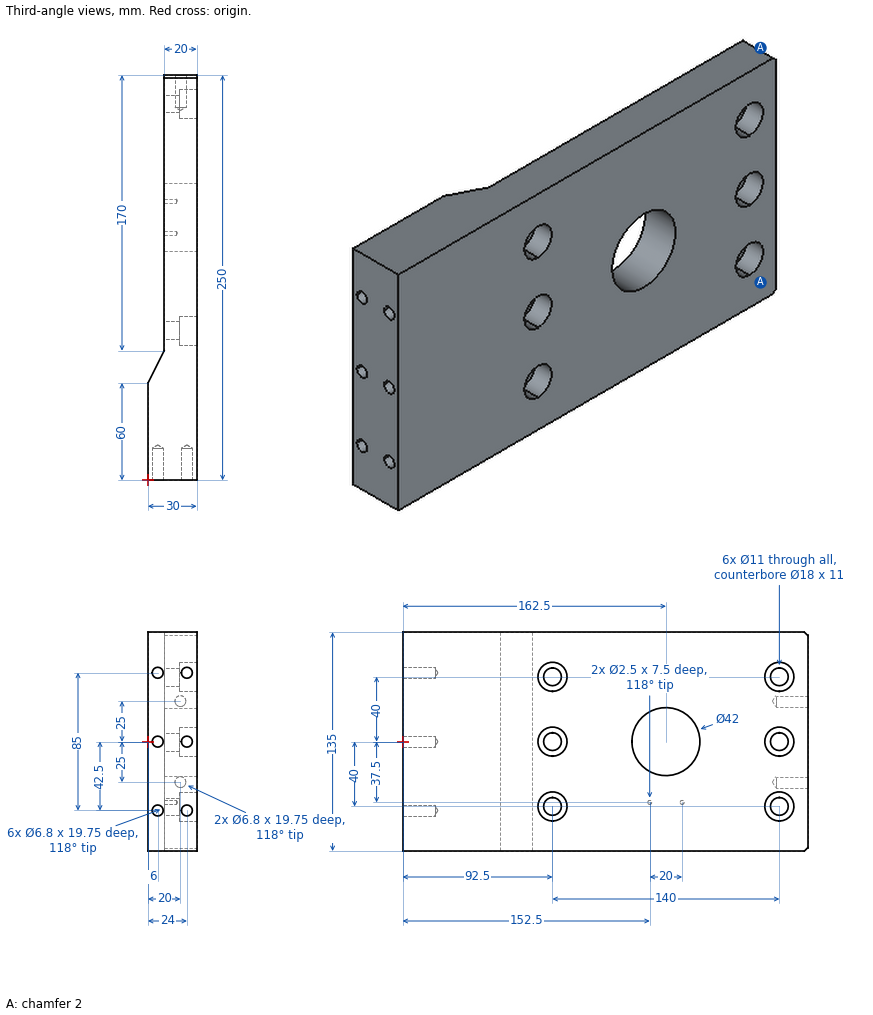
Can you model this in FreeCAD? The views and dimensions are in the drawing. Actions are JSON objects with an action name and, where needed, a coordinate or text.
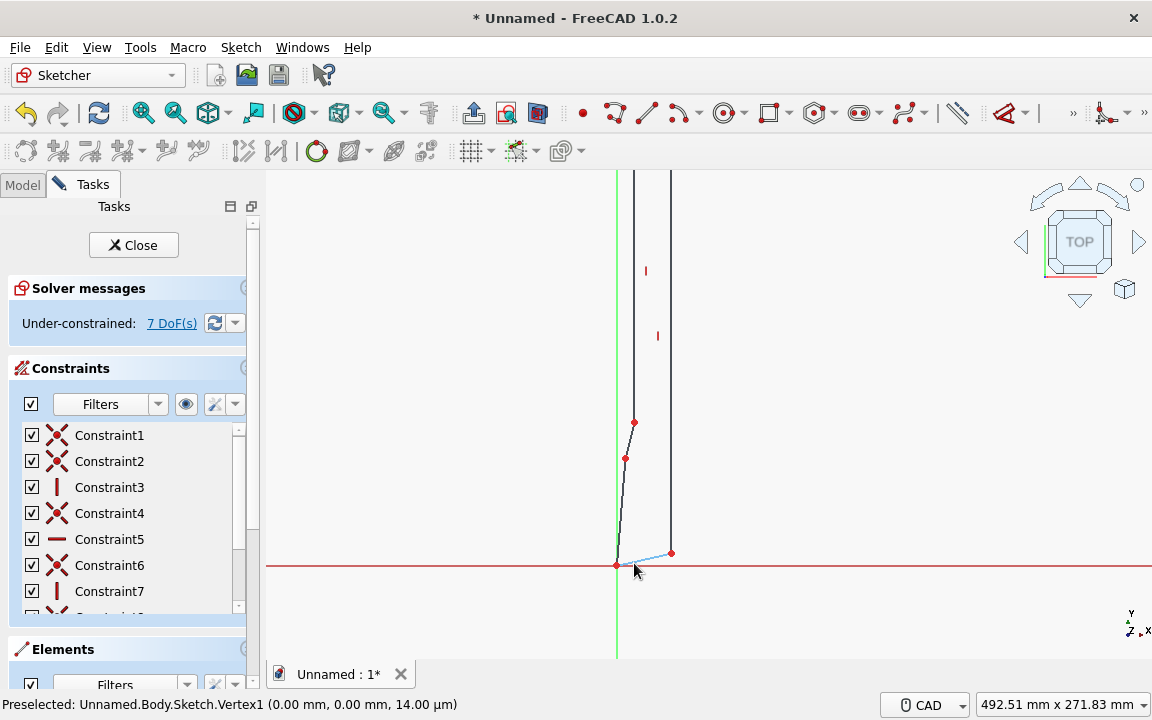
{"action": "left_click", "coordinate": [633, 562]}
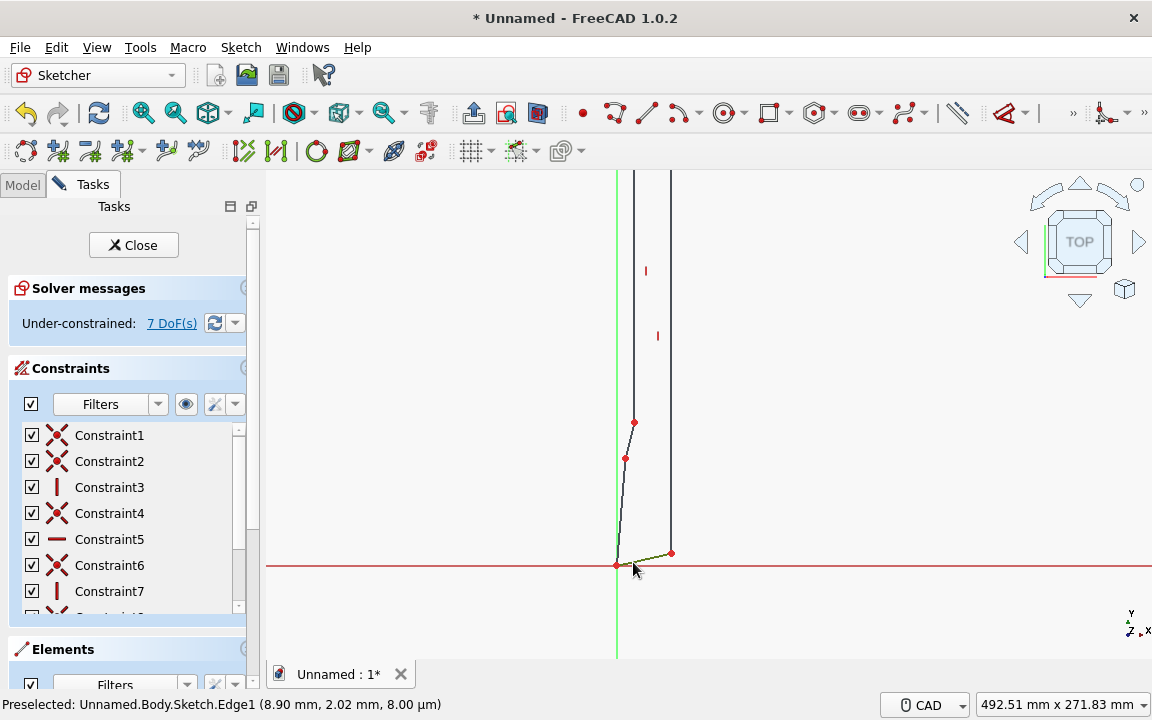
{"action": "key", "text": "h"}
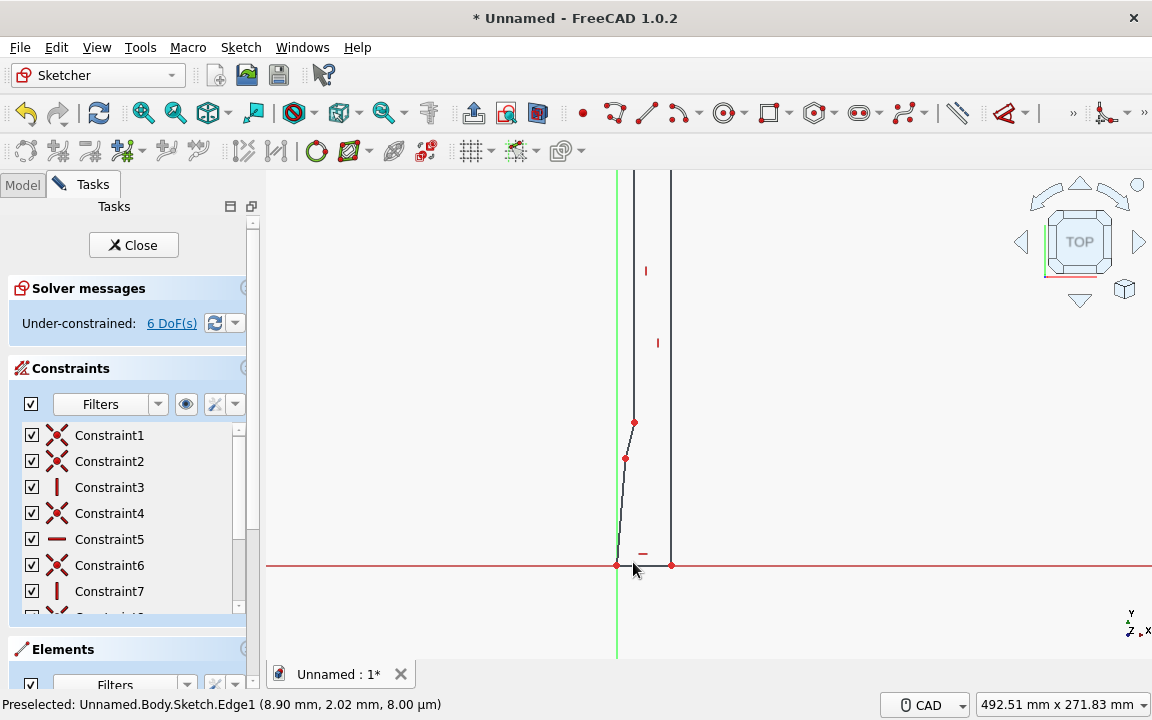
{"action": "left_click", "coordinate": [619, 534]}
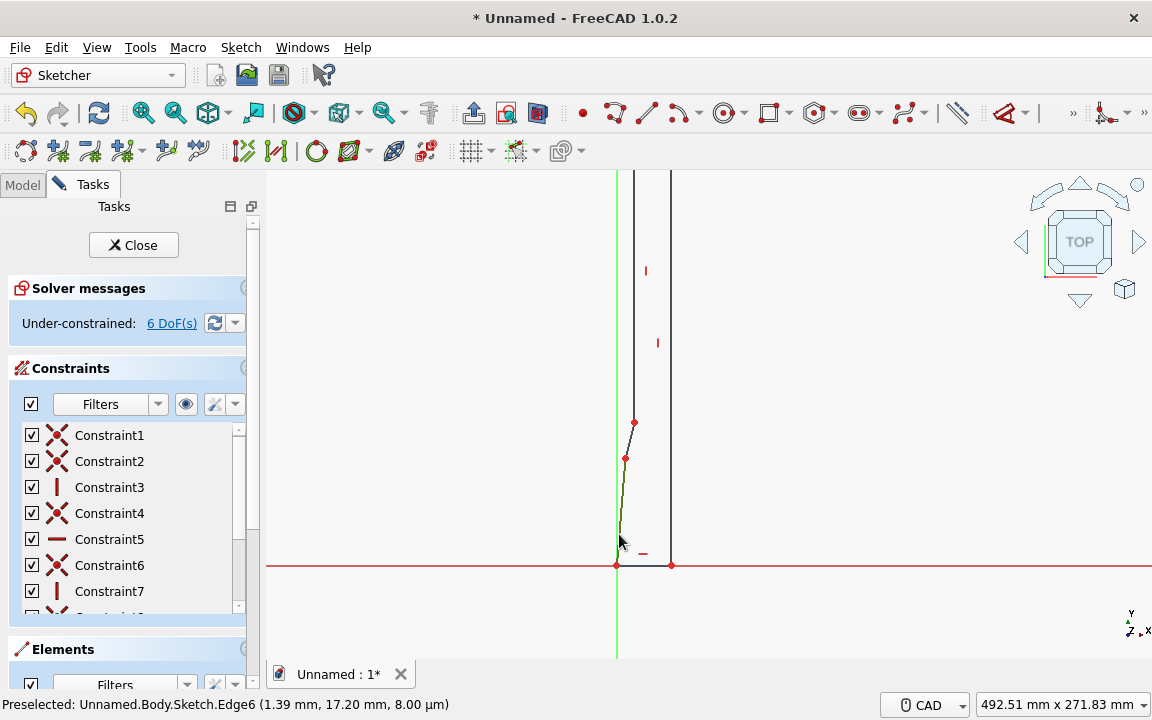
{"action": "key", "text": "v"}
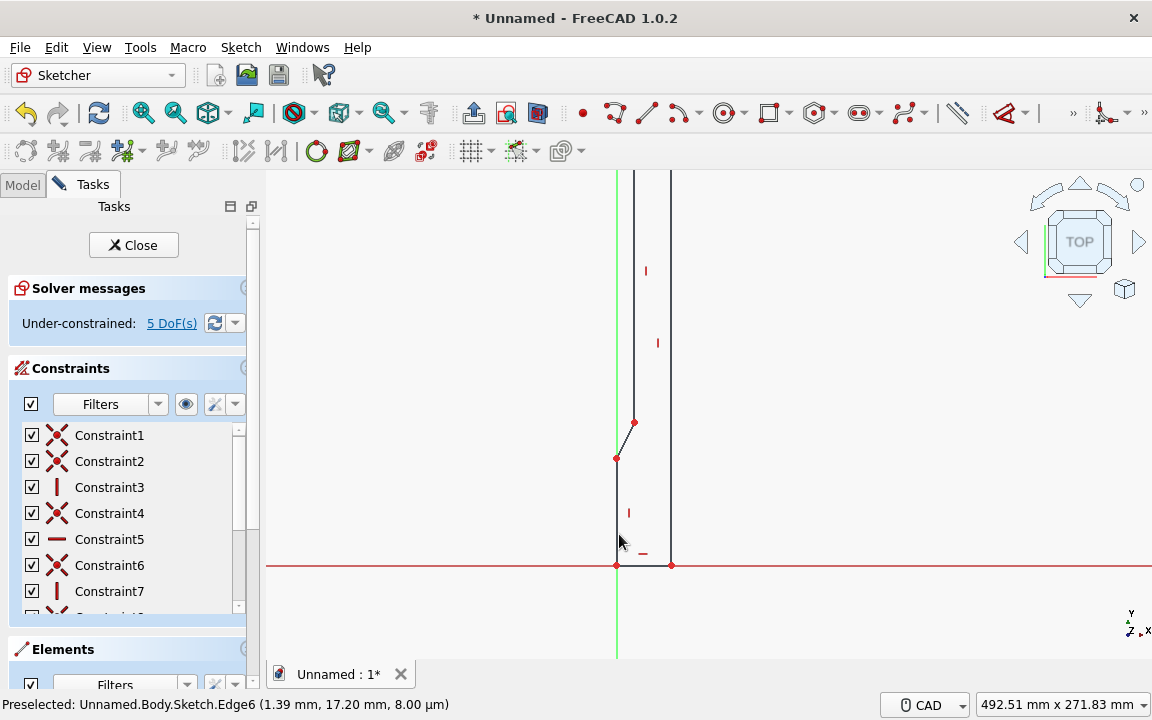
{"action": "left_click", "coordinate": [1004, 114]}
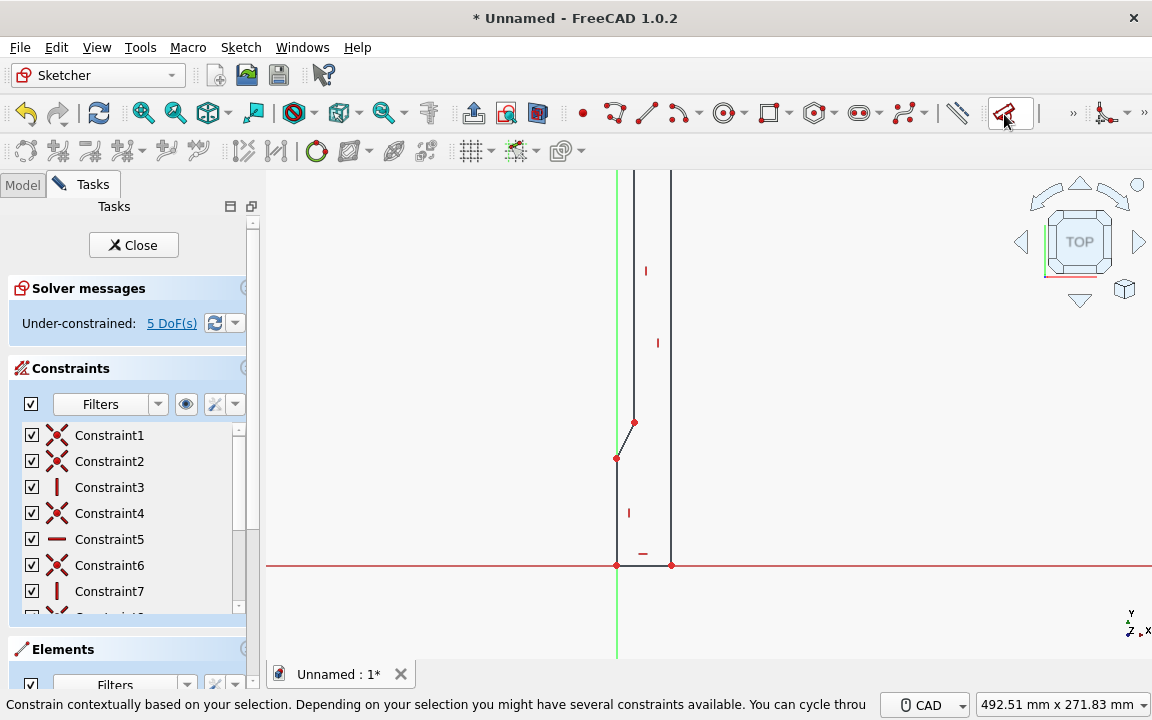
{"action": "left_click", "coordinate": [633, 566]}
{"action": "left_click", "coordinate": [644, 600]}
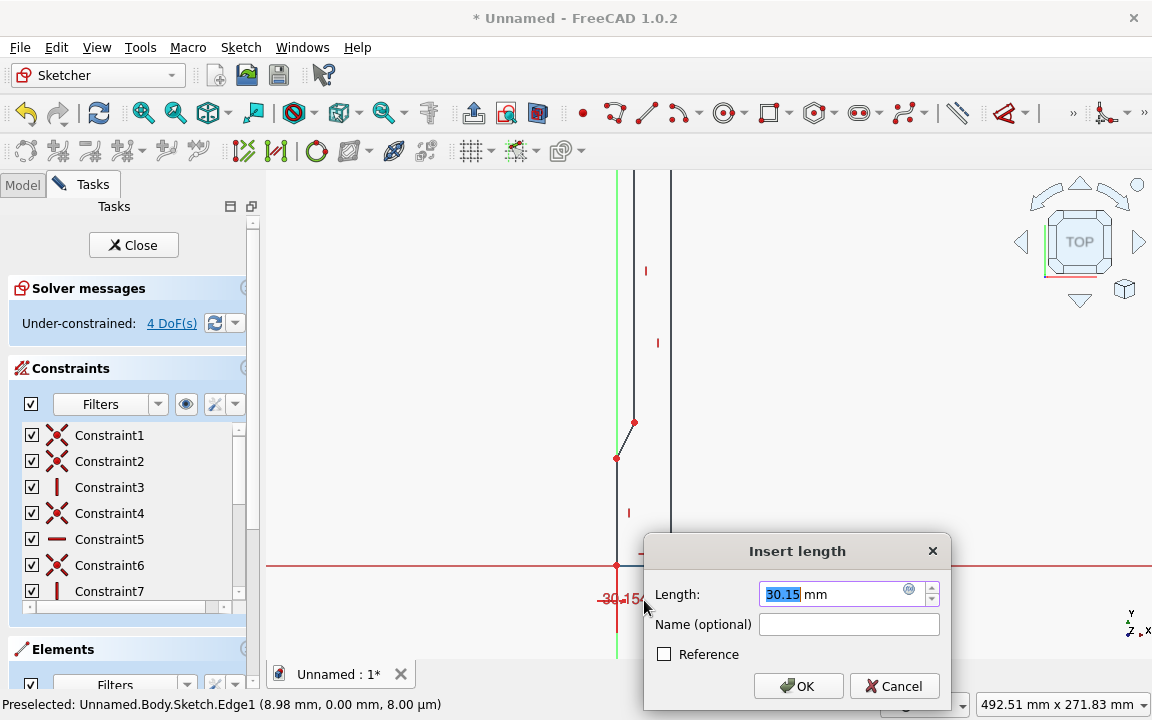
{"action": "type", "text": "30"}
{"action": "key", "text": "Return"}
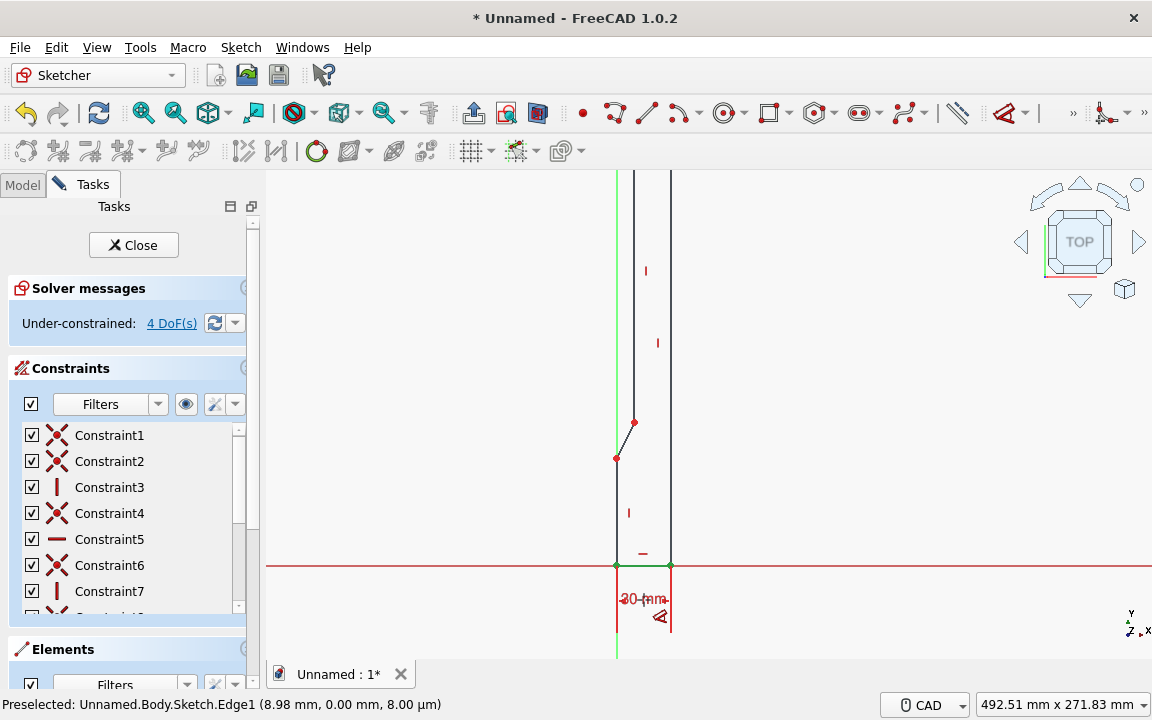
{"action": "scroll", "coordinate": [634, 564], "scroll_direction": "down", "scroll_amount": 2}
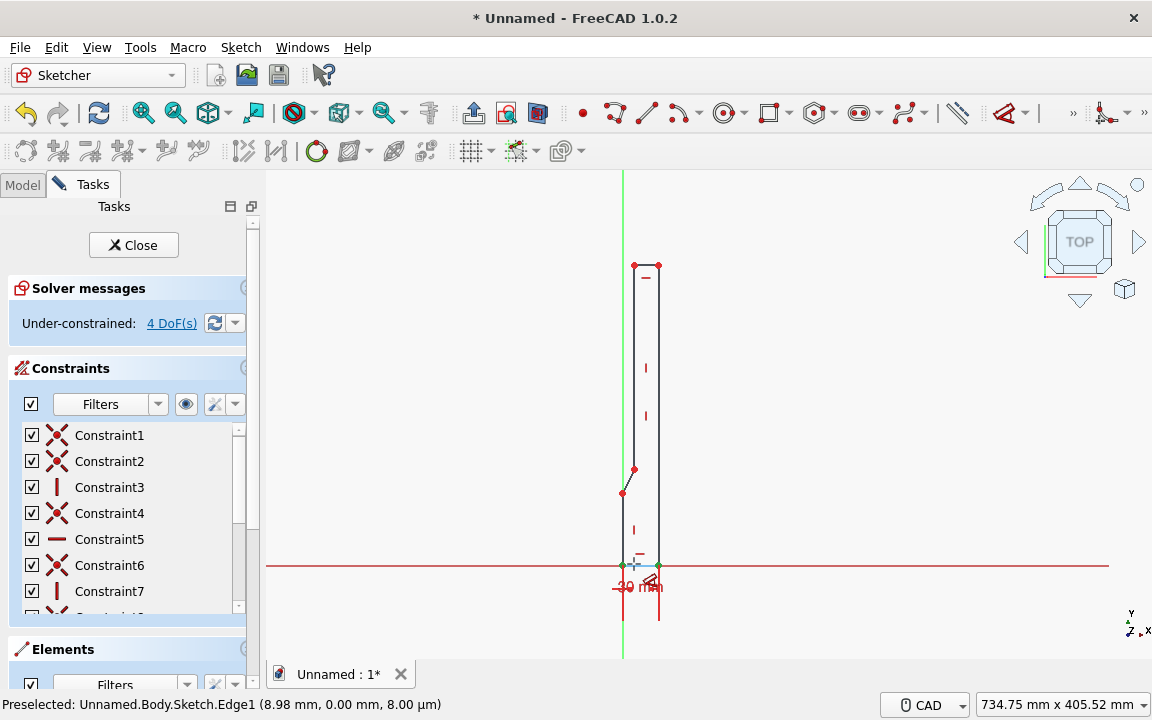
{"action": "scroll", "coordinate": [652, 265], "scroll_direction": "up", "scroll_amount": 4}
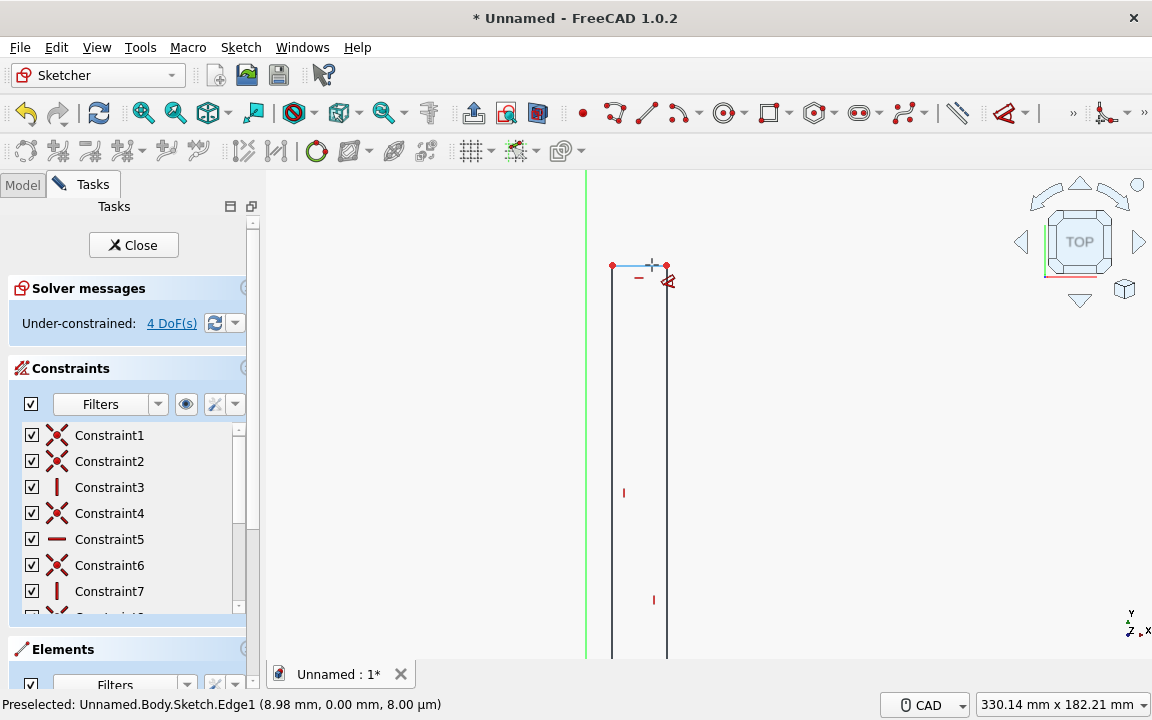
{"action": "left_click", "coordinate": [650, 266]}
{"action": "left_click", "coordinate": [640, 232]}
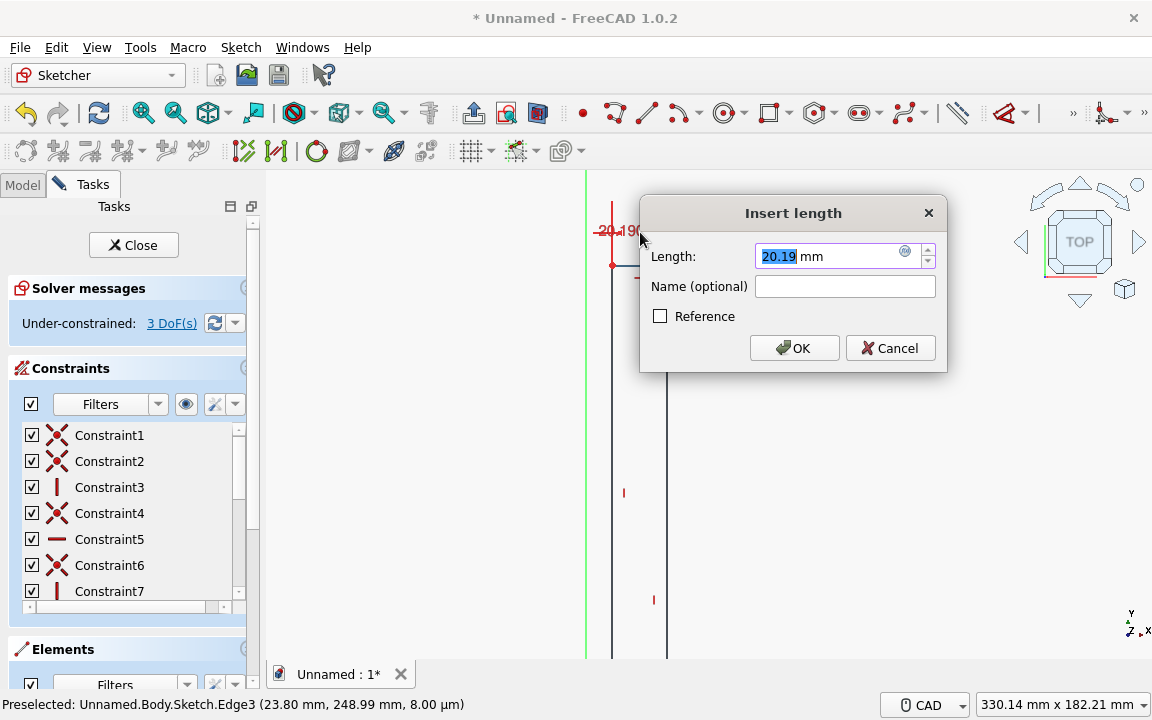
{"action": "type", "text": "20"}
{"action": "key", "text": "Return"}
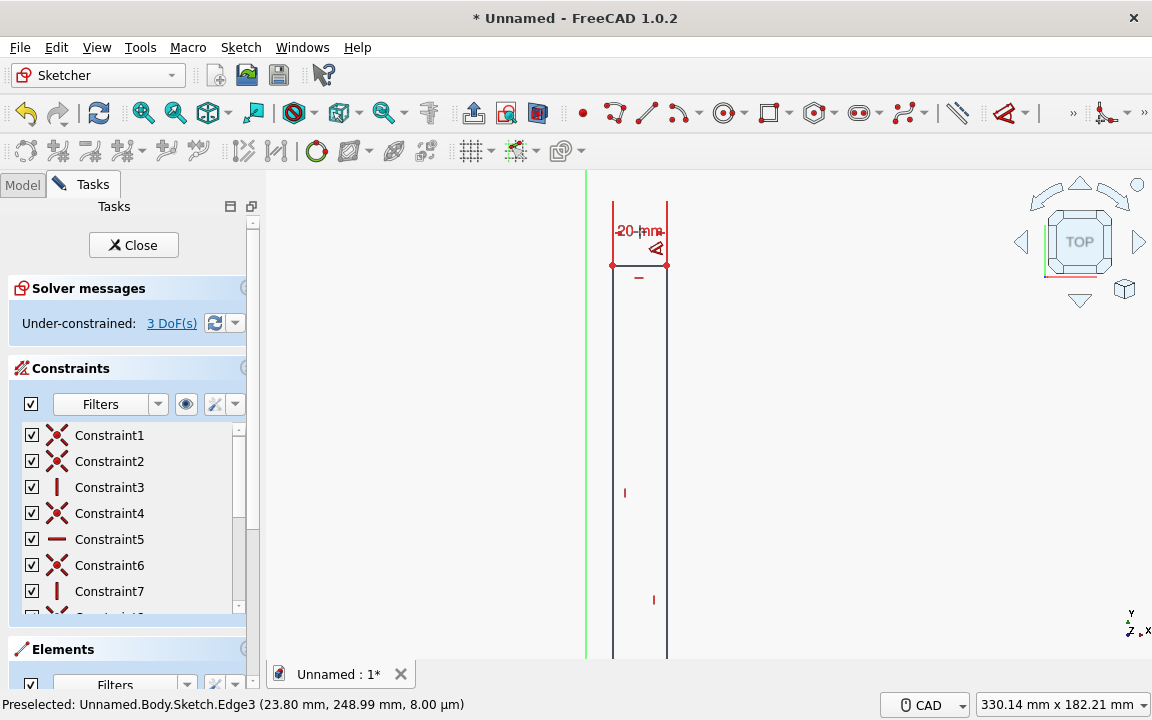
{"action": "scroll", "coordinate": [652, 265], "scroll_direction": "down", "scroll_amount": 4}